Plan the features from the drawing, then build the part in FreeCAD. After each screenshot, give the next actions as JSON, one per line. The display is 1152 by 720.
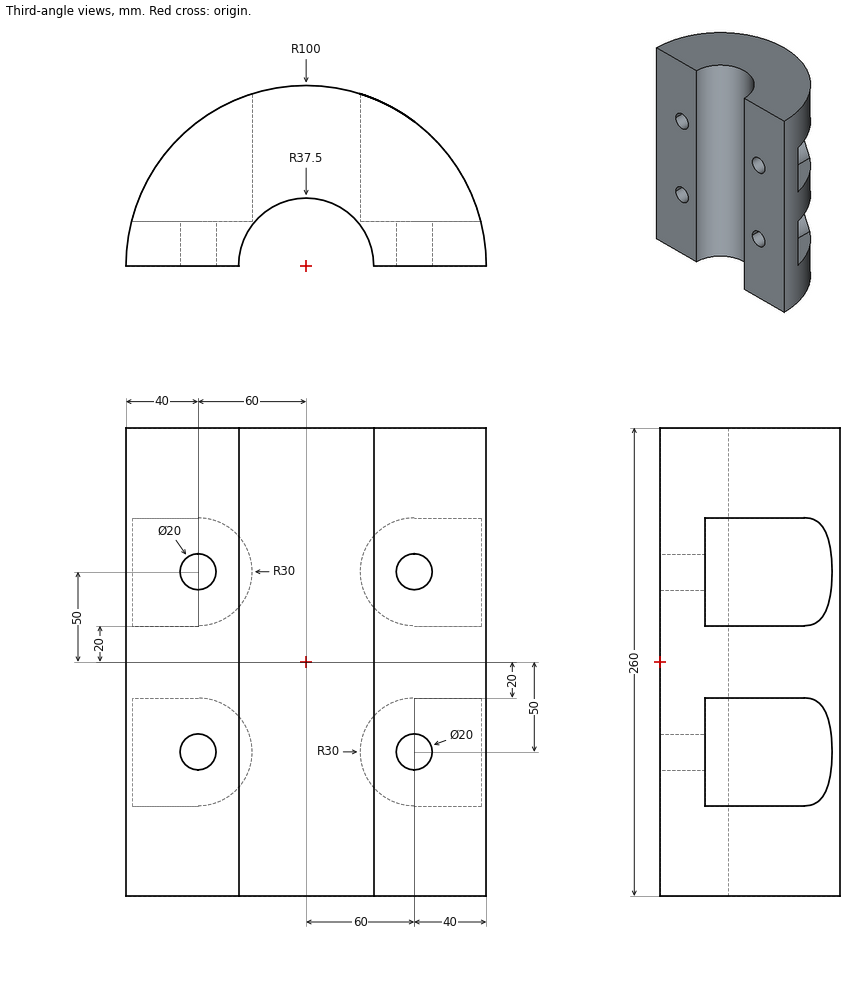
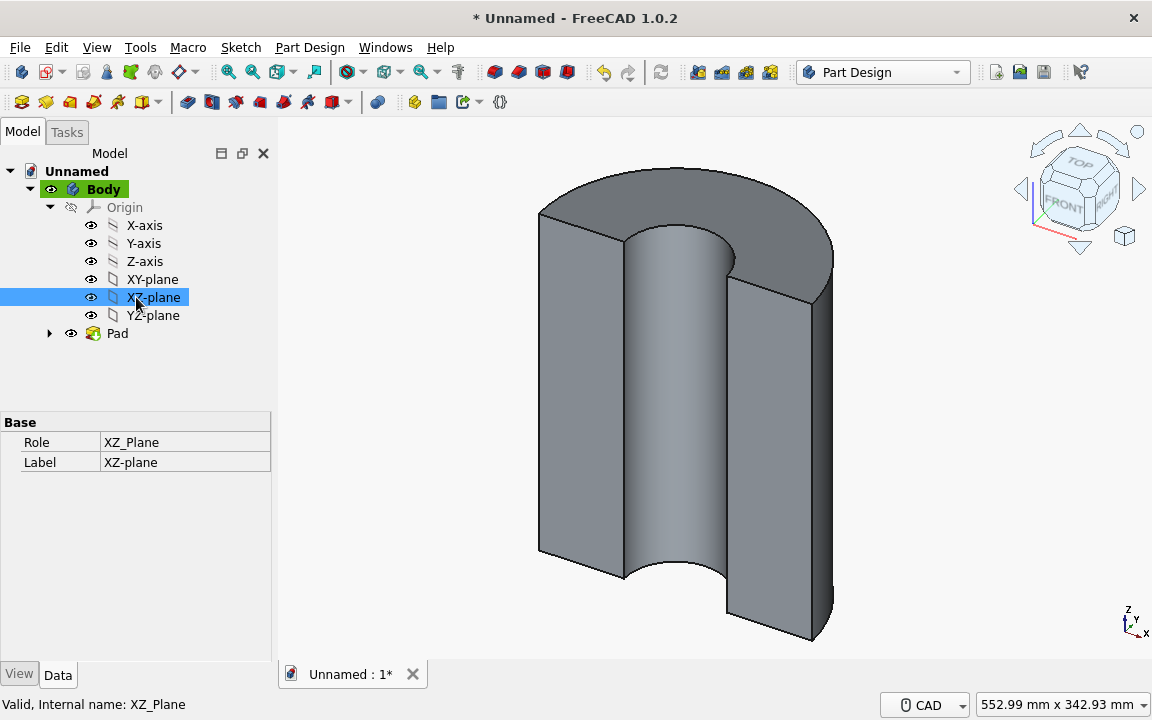
{"action": "left_click", "coordinate": [180, 72]}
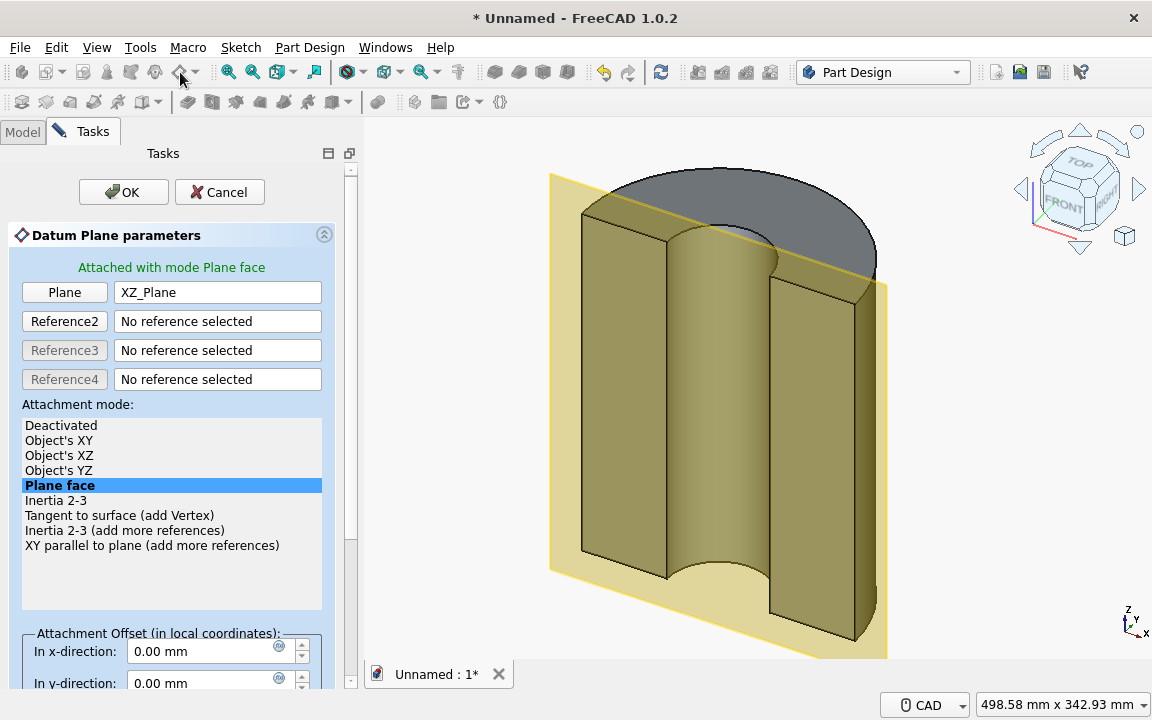
{"action": "scroll", "coordinate": [351, 426], "scroll_direction": "down", "scroll_amount": 2}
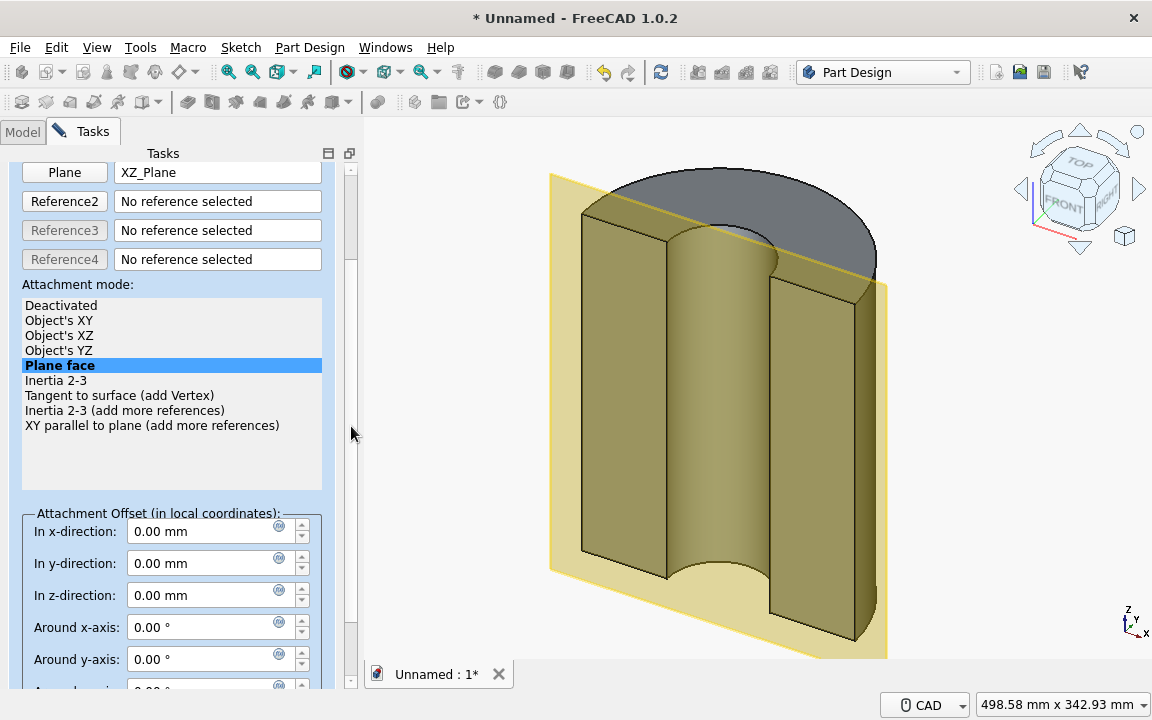
{"action": "triple_click", "coordinate": [210, 595]}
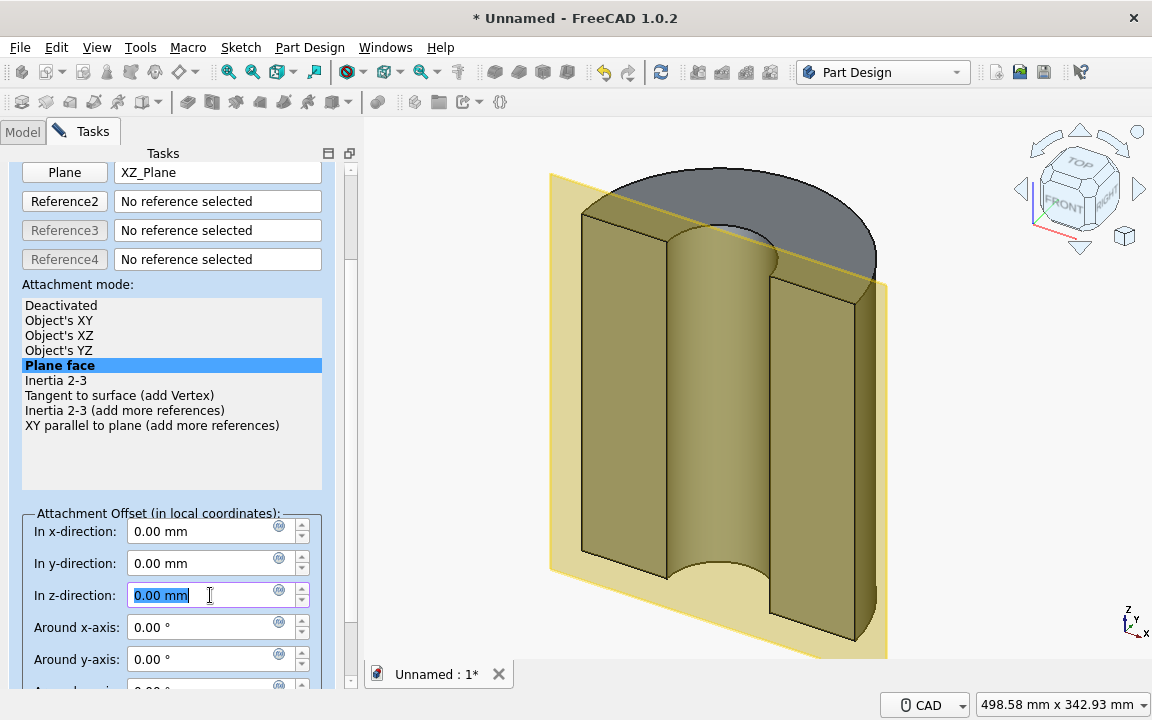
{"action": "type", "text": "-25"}
{"action": "key", "text": "Tab"}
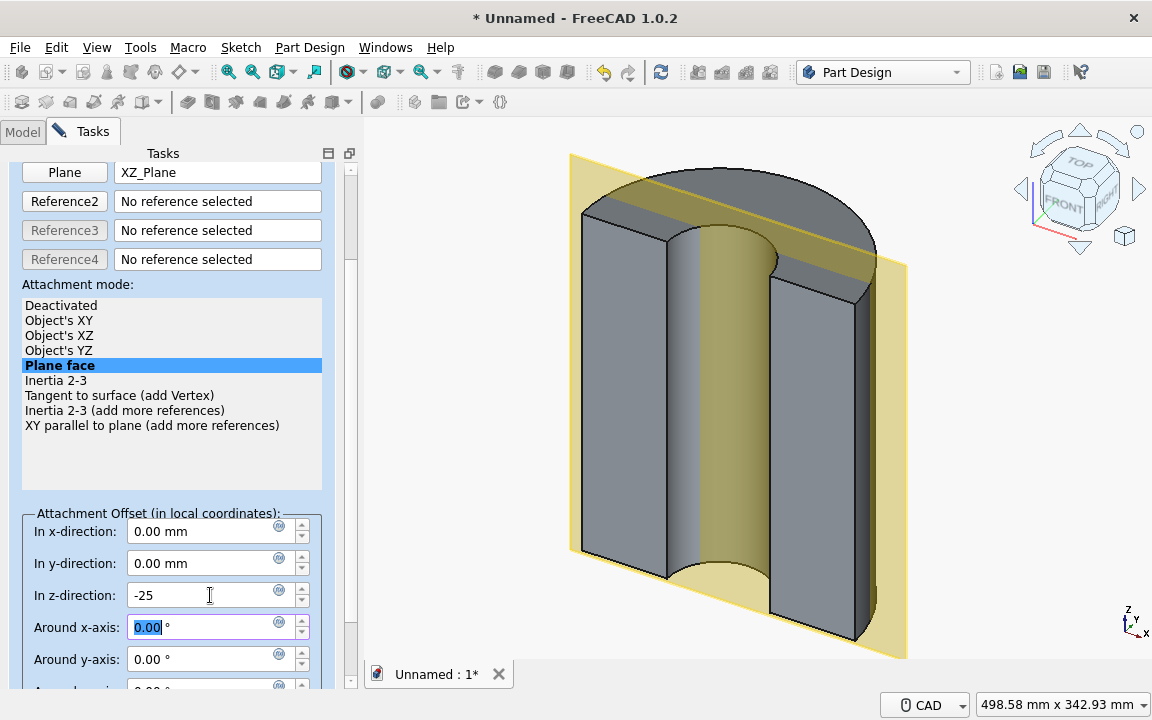
{"action": "scroll", "coordinate": [351, 426], "scroll_direction": "up", "scroll_amount": 3}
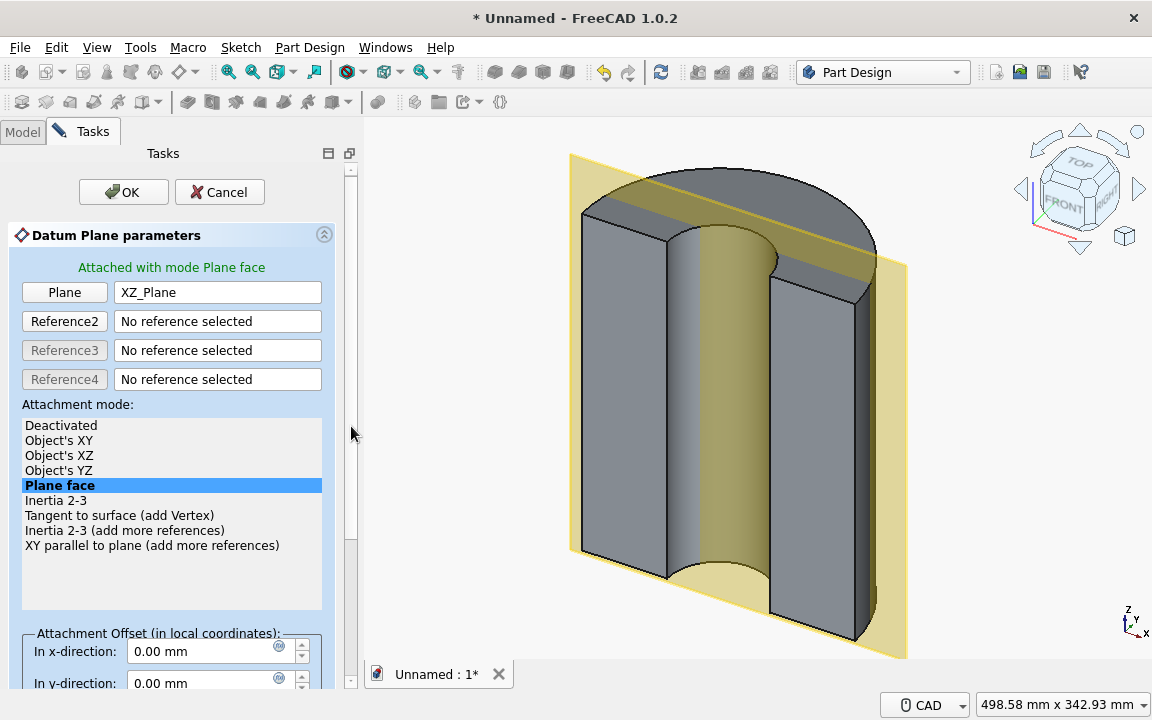
{"action": "left_click", "coordinate": [124, 192]}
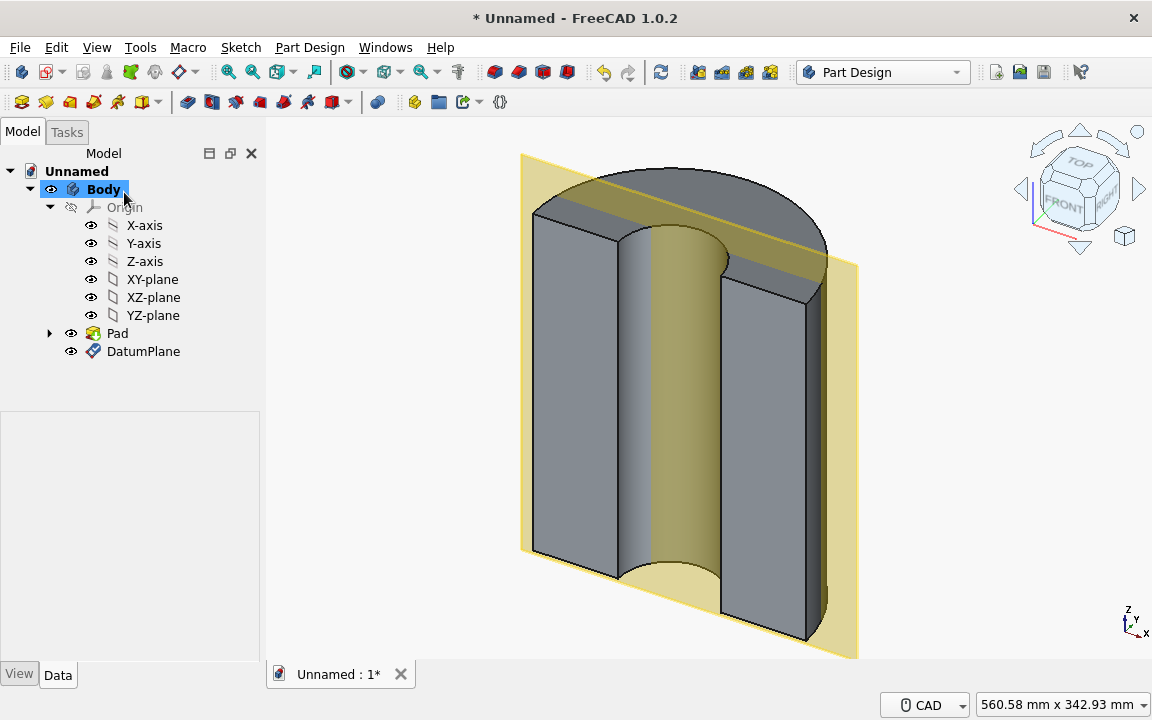
{"action": "left_click", "coordinate": [116, 351]}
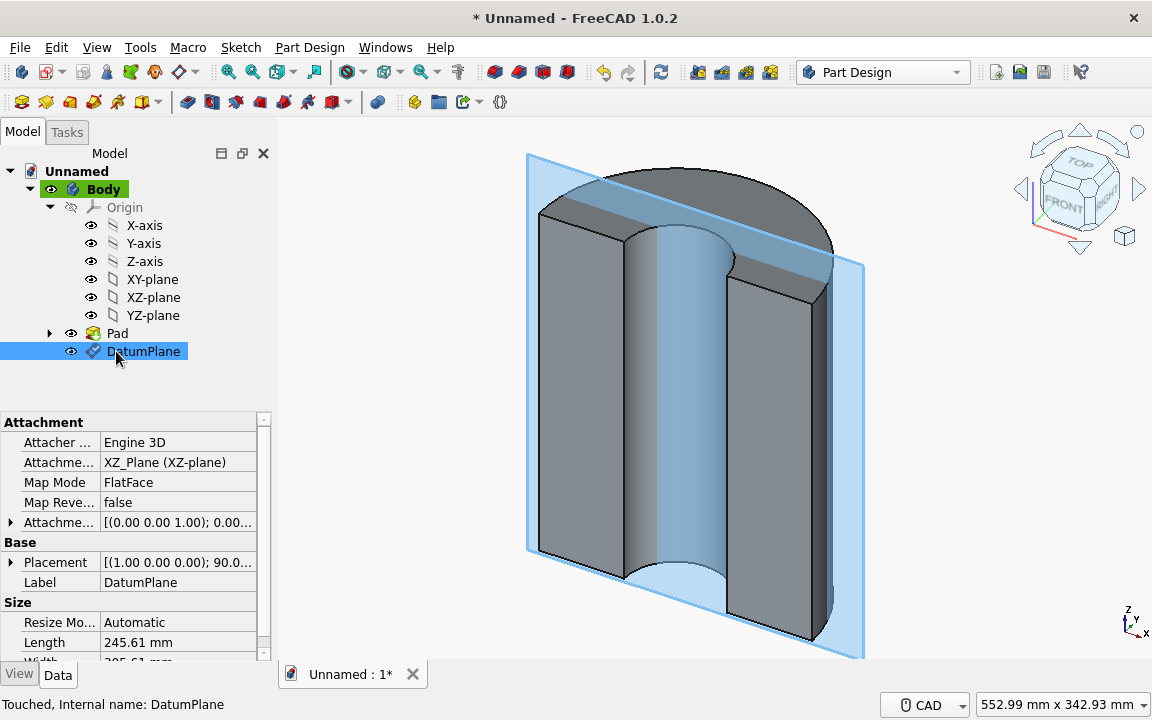
{"action": "left_click", "coordinate": [46, 72]}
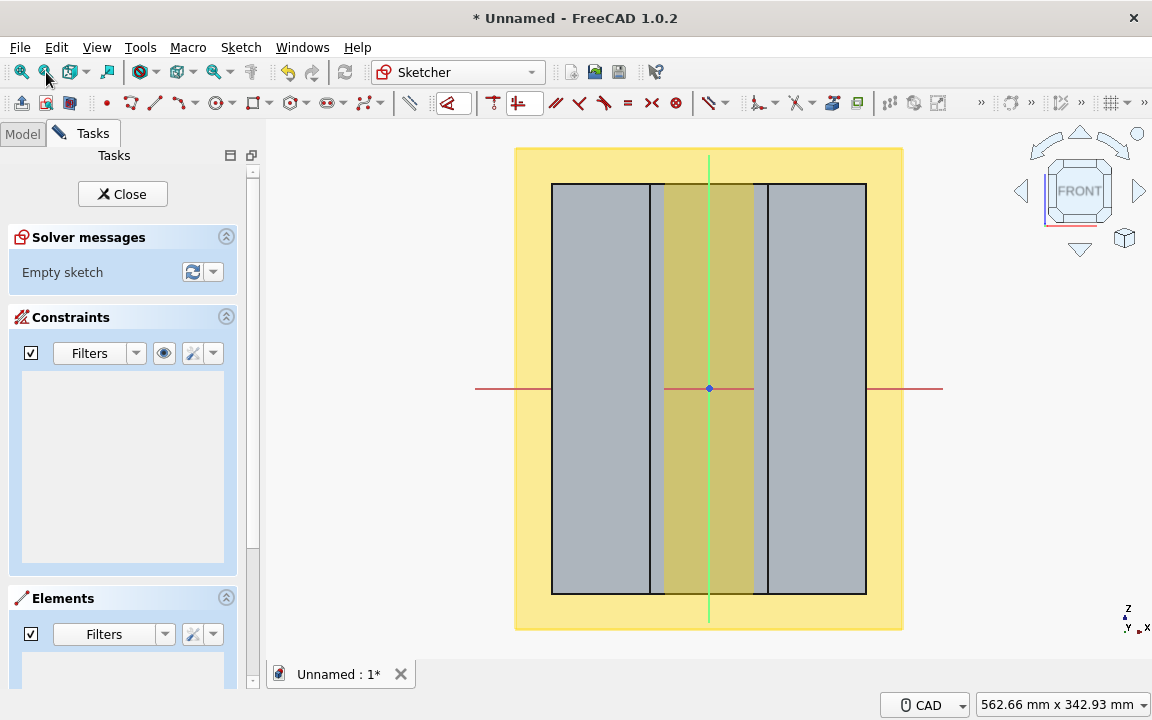
{"action": "left_click", "coordinate": [70, 104]}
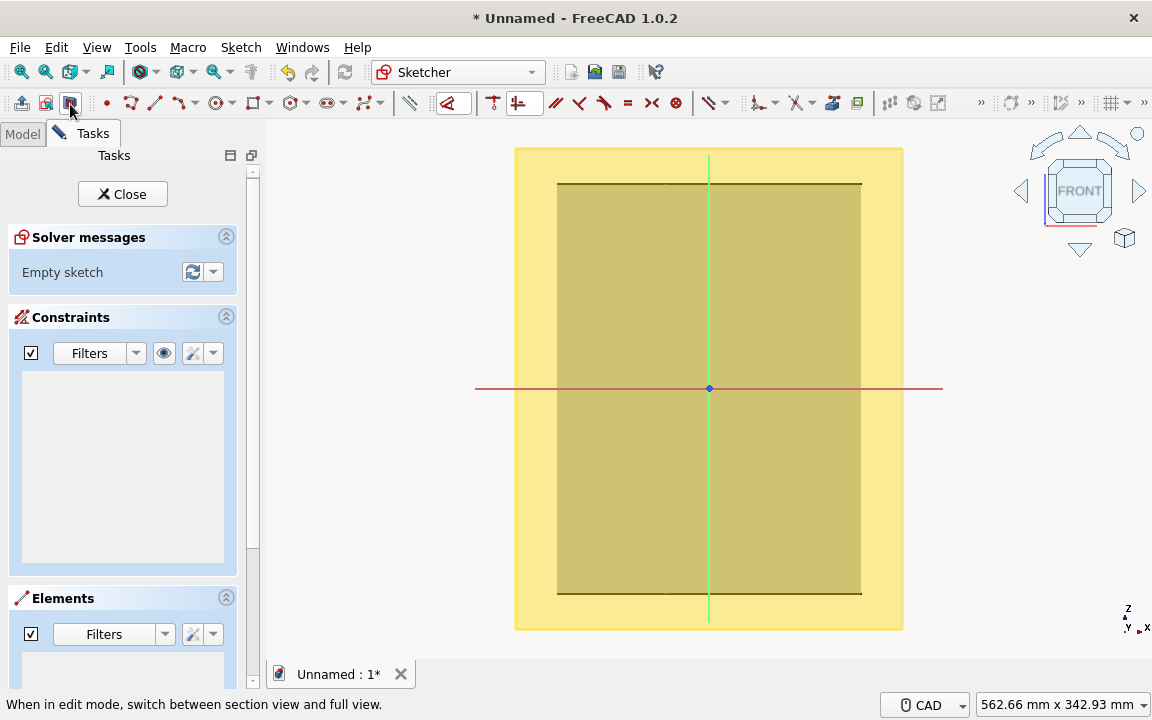
{"action": "scroll", "coordinate": [624, 289], "scroll_direction": "up", "scroll_amount": 5}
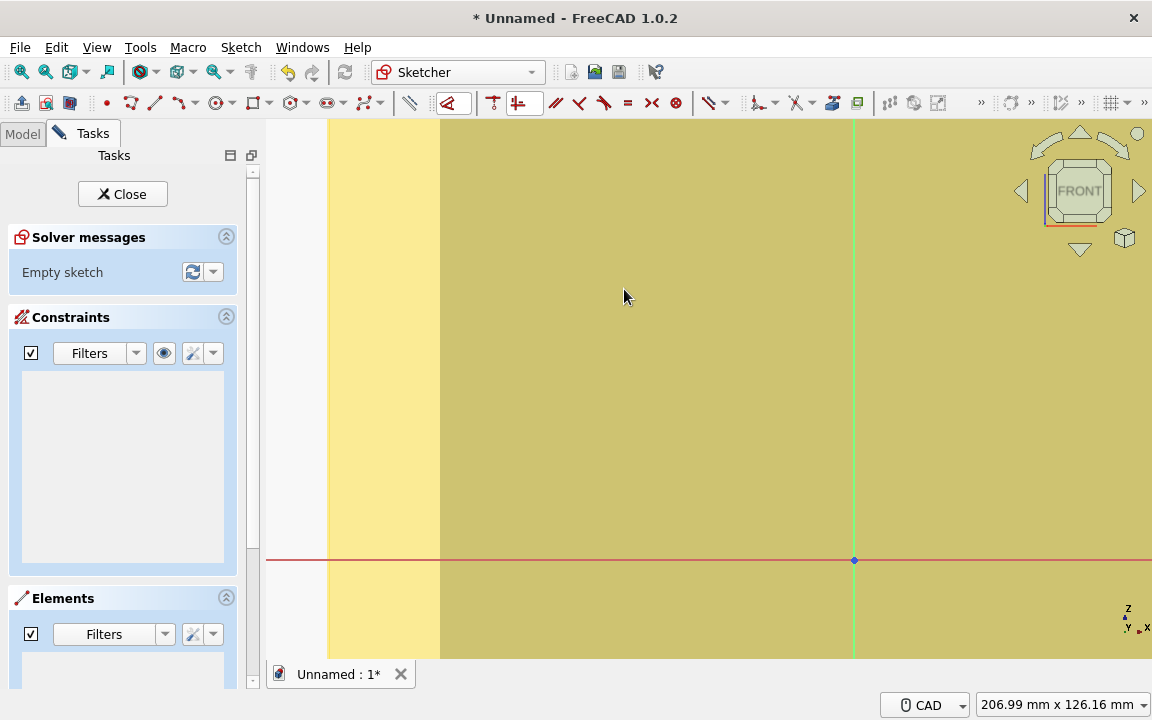
{"action": "left_click", "coordinate": [132, 104]}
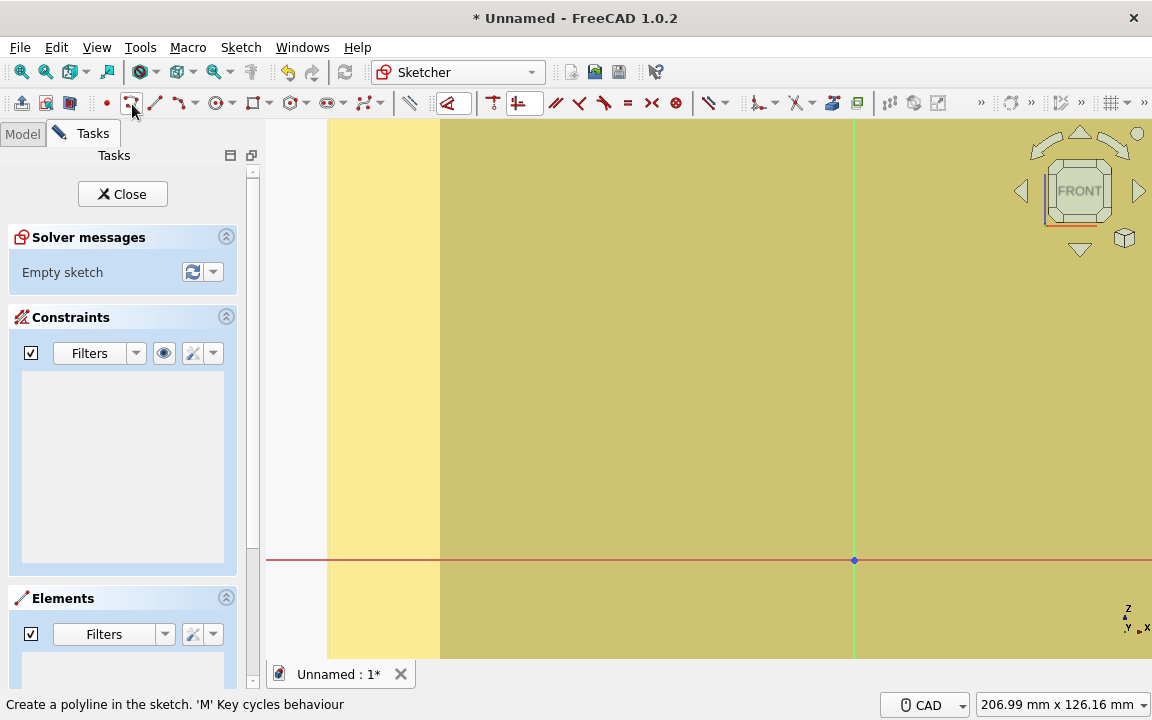
{"action": "left_click", "coordinate": [598, 475]}
{"action": "left_click", "coordinate": [426, 475]}
{"action": "left_click", "coordinate": [426, 218]}
{"action": "left_click", "coordinate": [598, 218]}
{"action": "right_click", "coordinate": [598, 218]}